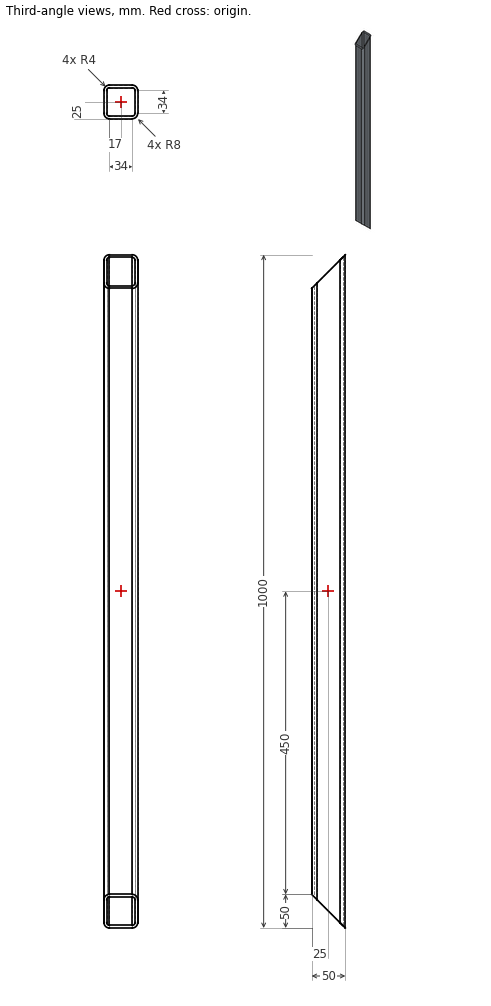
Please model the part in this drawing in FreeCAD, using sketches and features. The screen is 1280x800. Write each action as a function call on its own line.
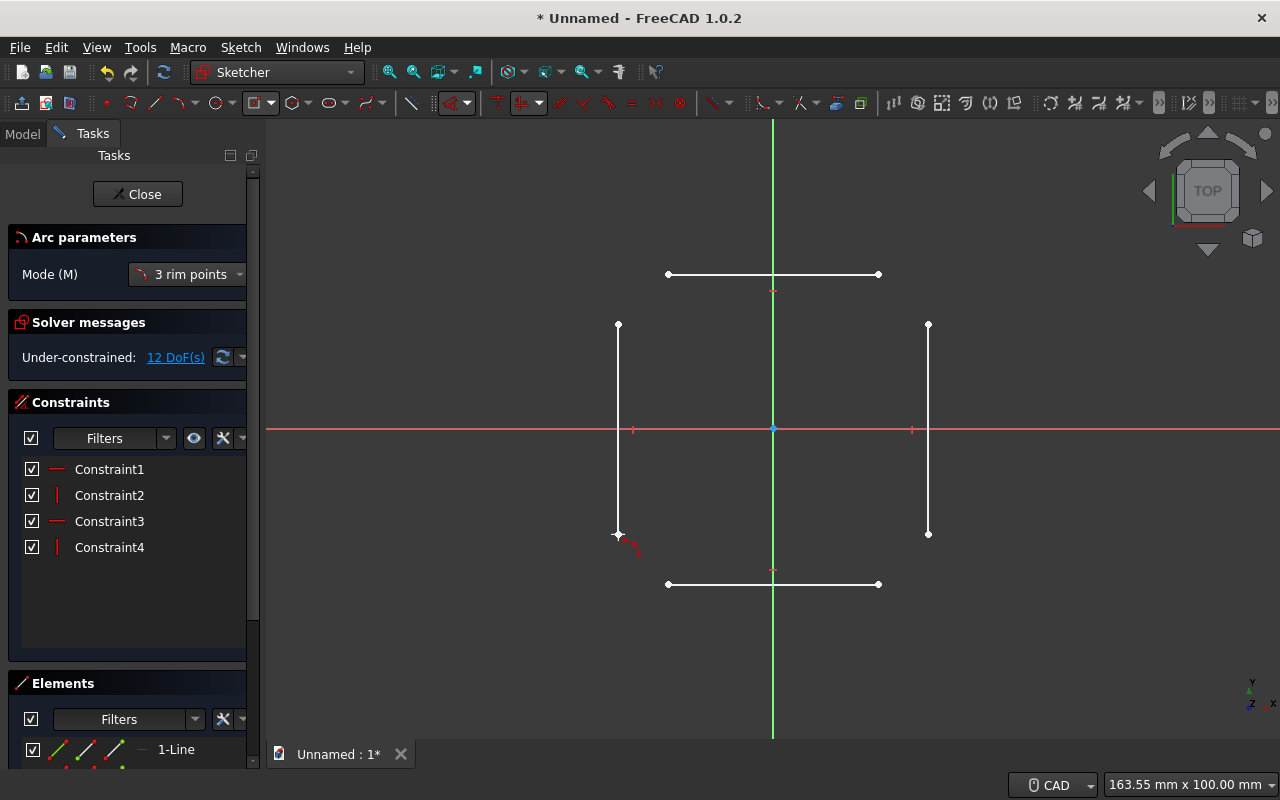
click(878, 585)
click(928, 535)
click(913, 569)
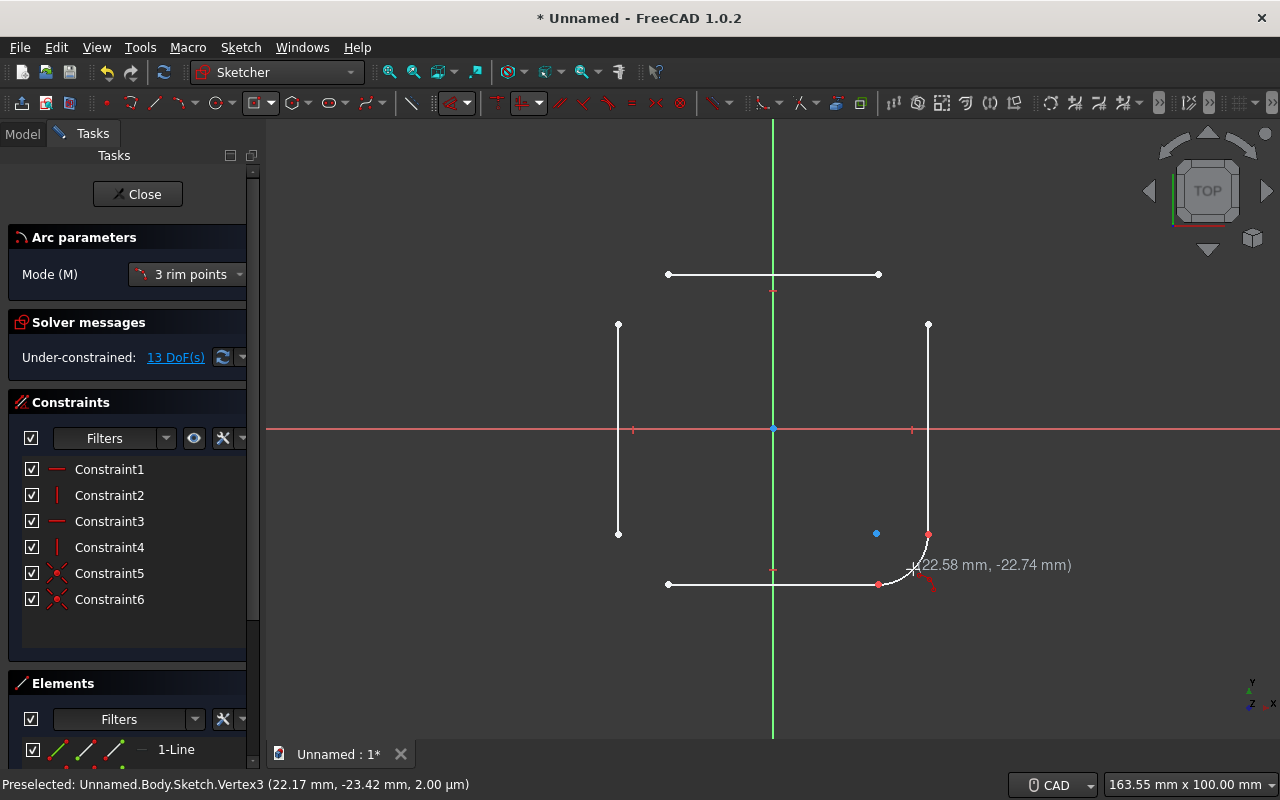
click(928, 325)
click(878, 275)
click(913, 289)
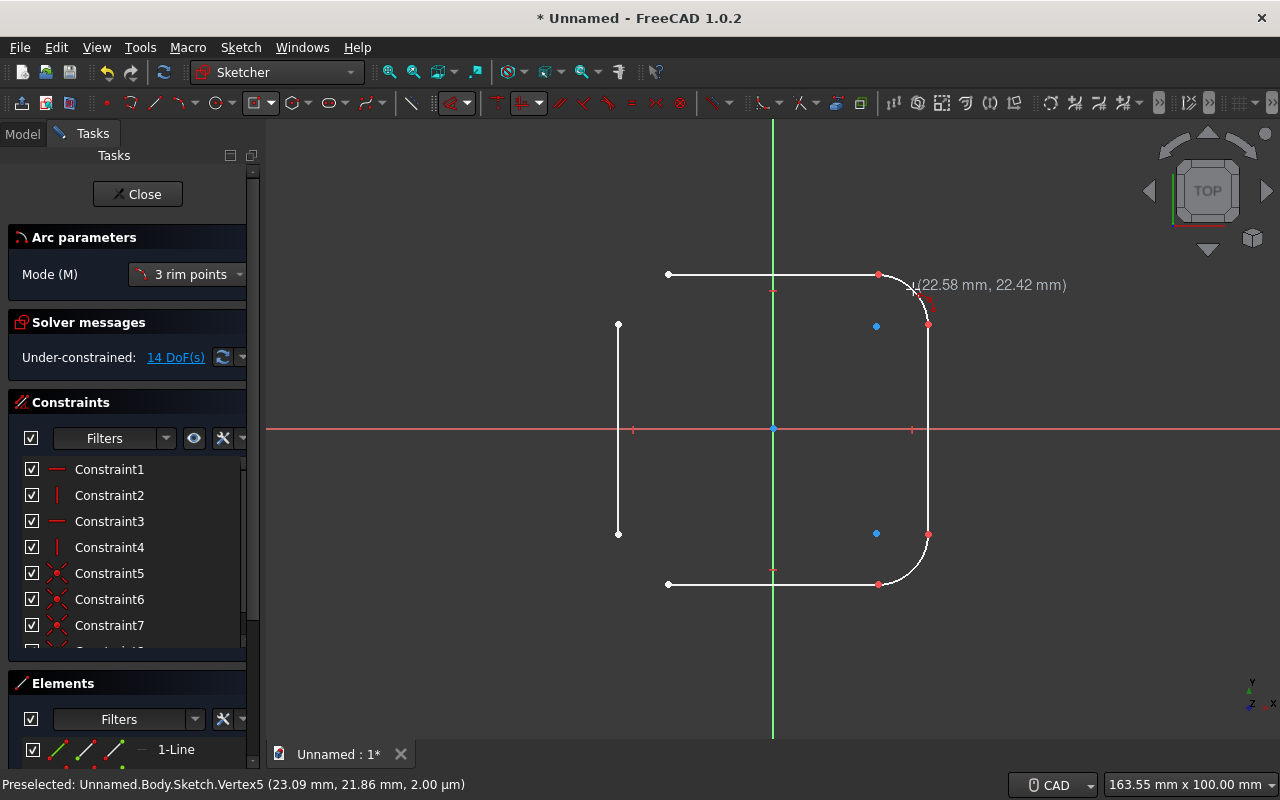
click(668, 275)
click(618, 325)
click(633, 289)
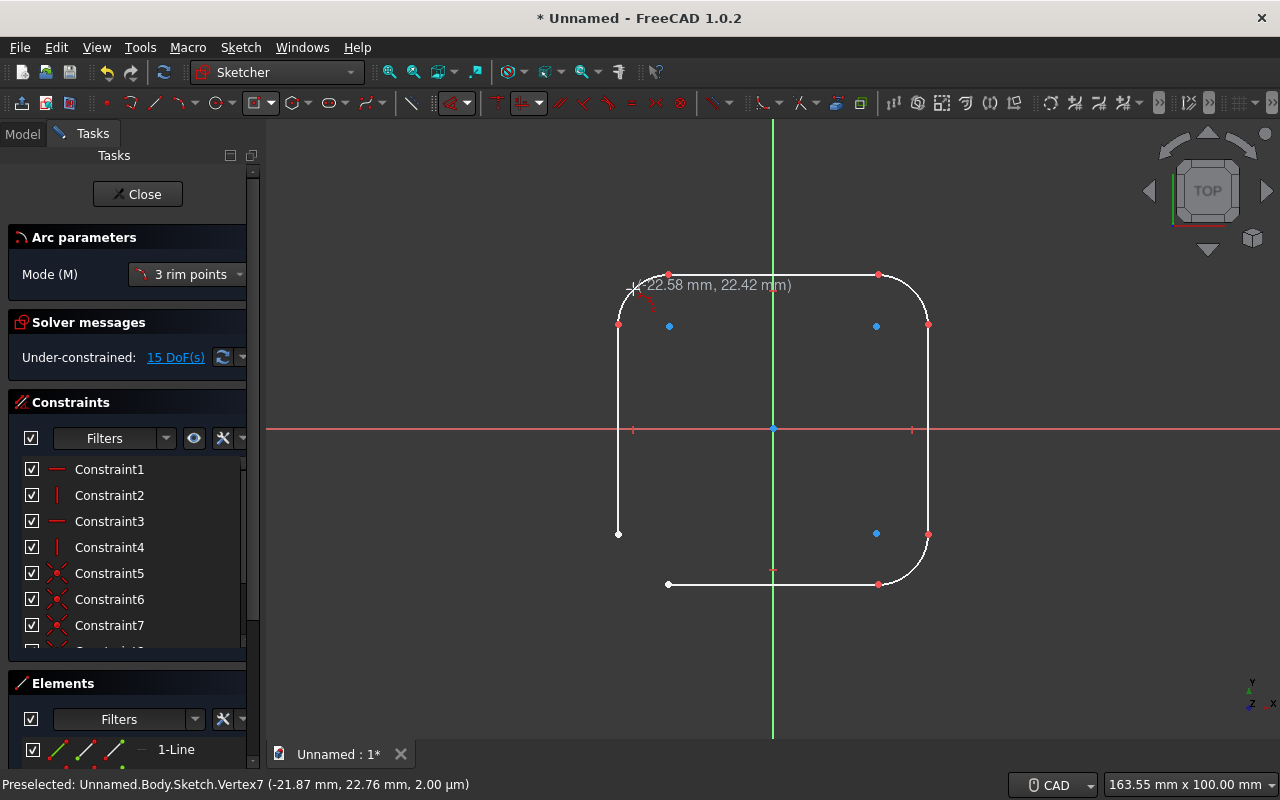
click(618, 535)
click(668, 585)
click(633, 569)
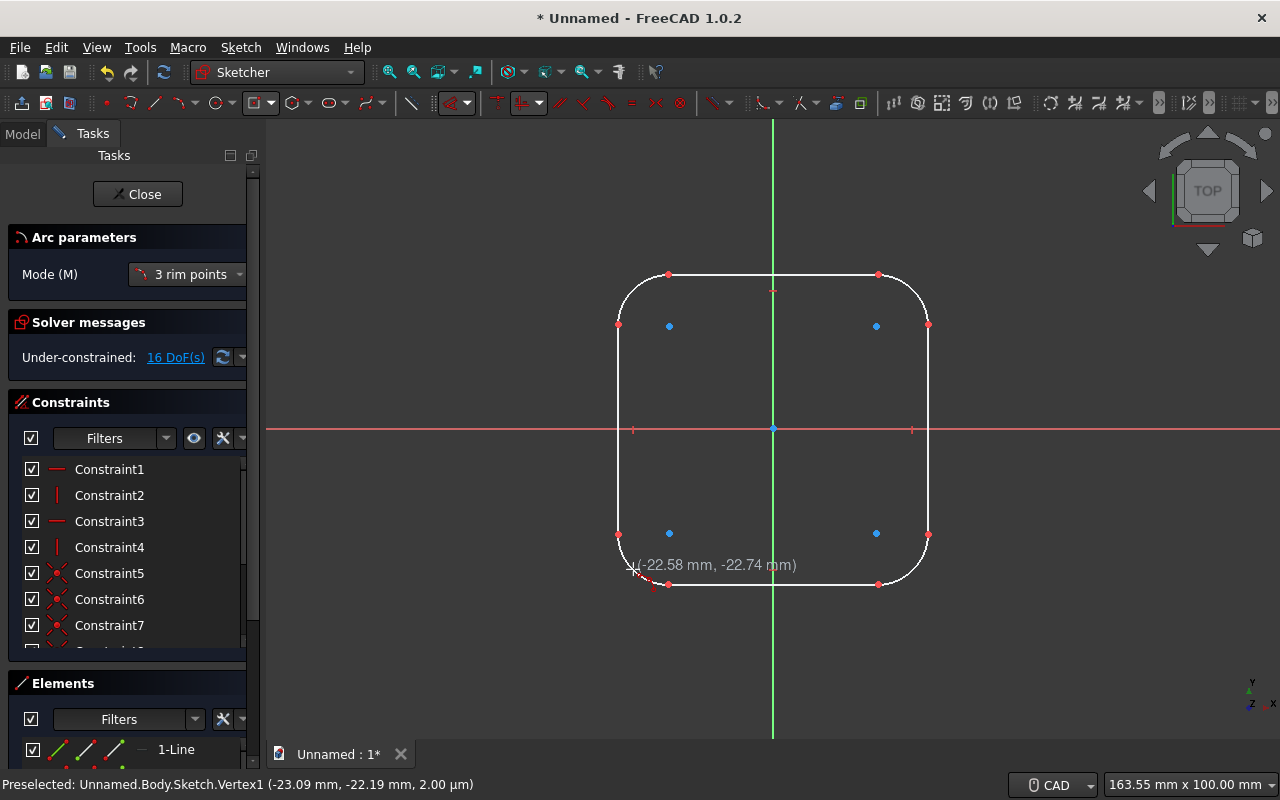
key(g)
key(l)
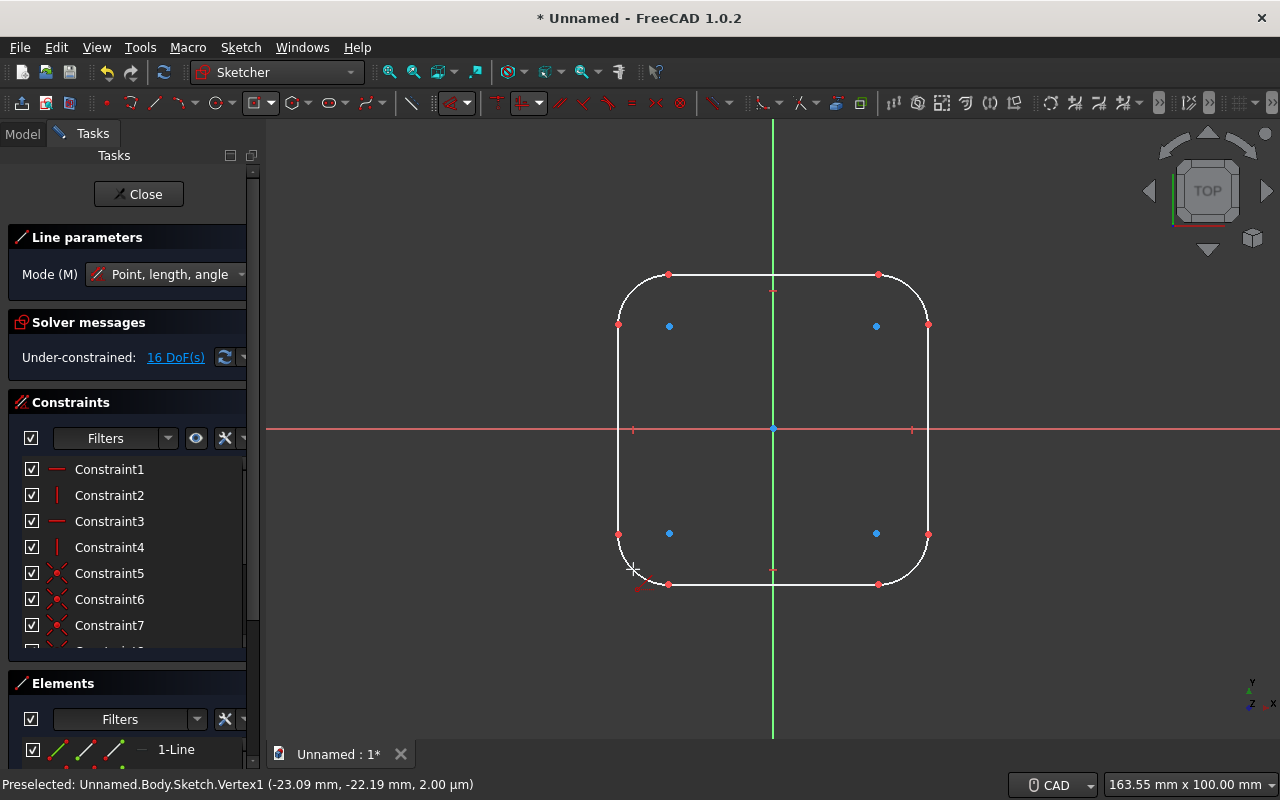
click(668, 299)
click(878, 299)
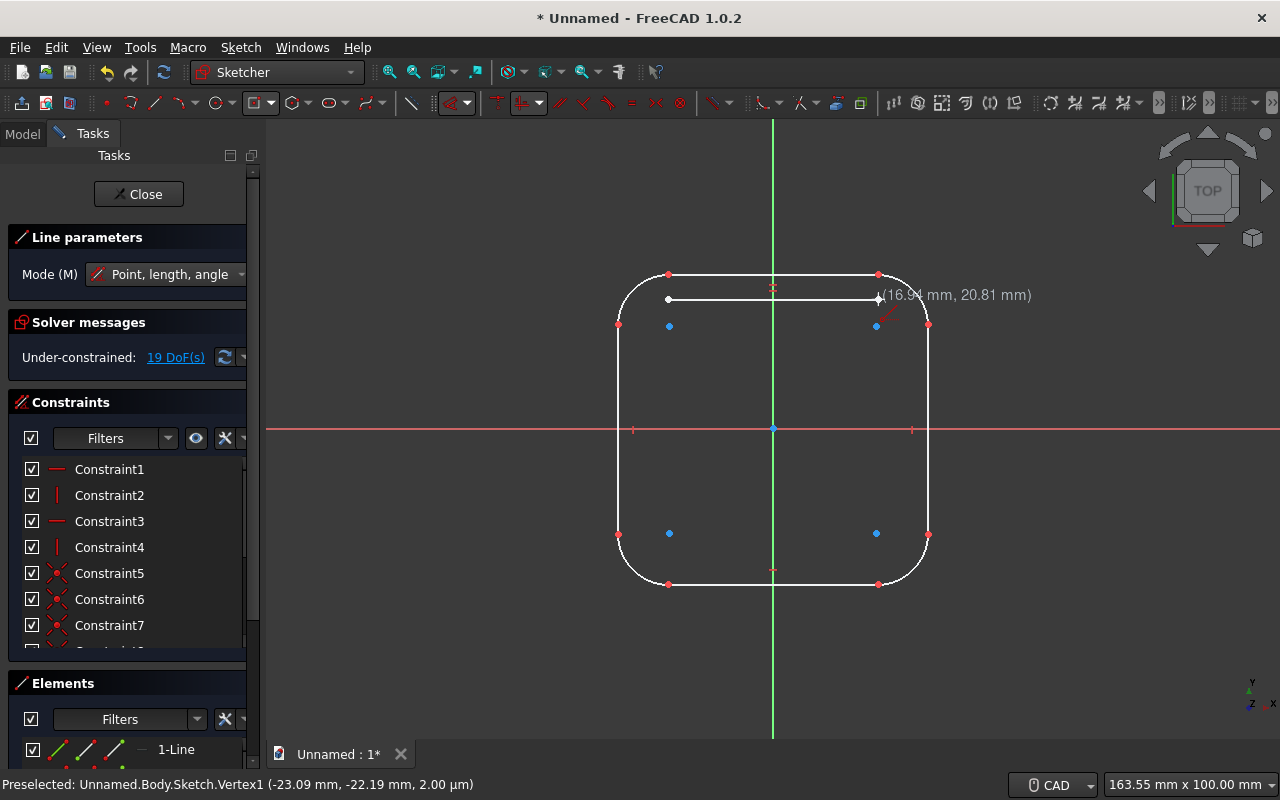
click(903, 324)
click(903, 534)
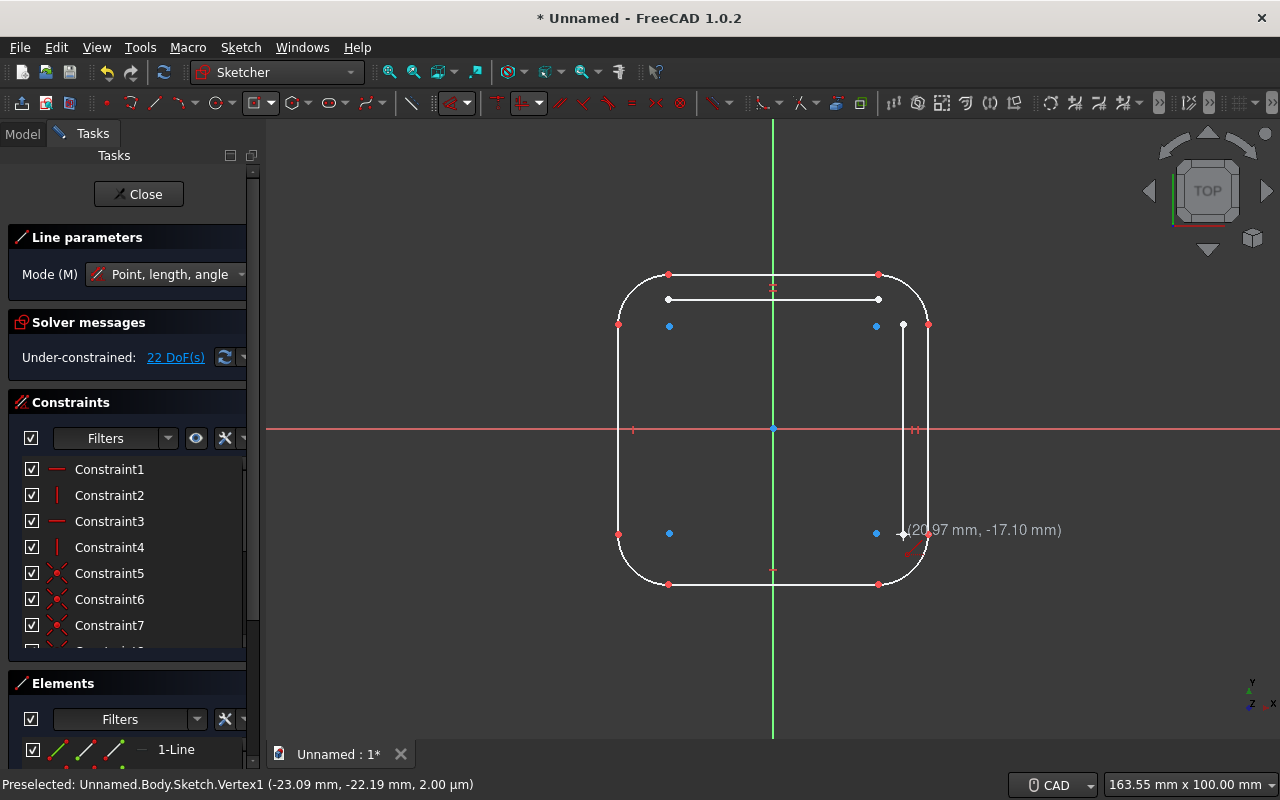
click(878, 559)
click(668, 559)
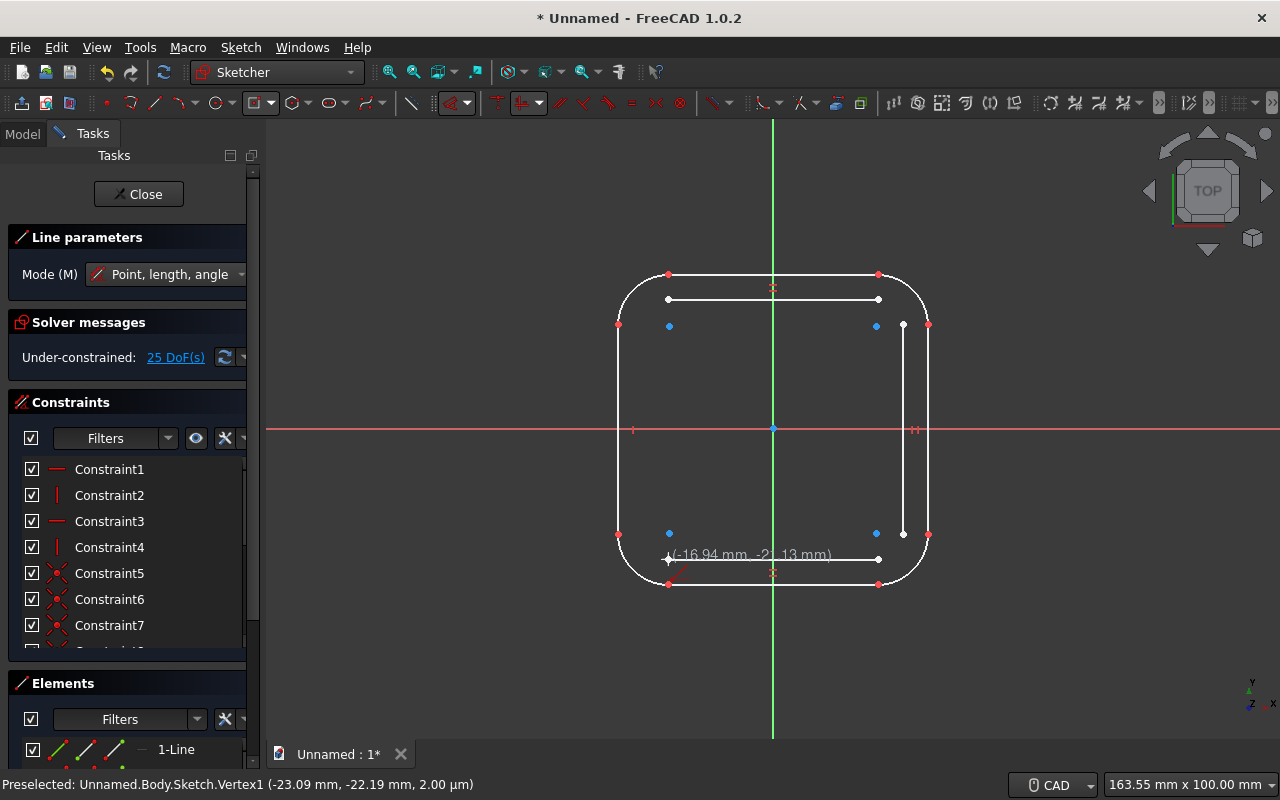
click(643, 534)
click(643, 324)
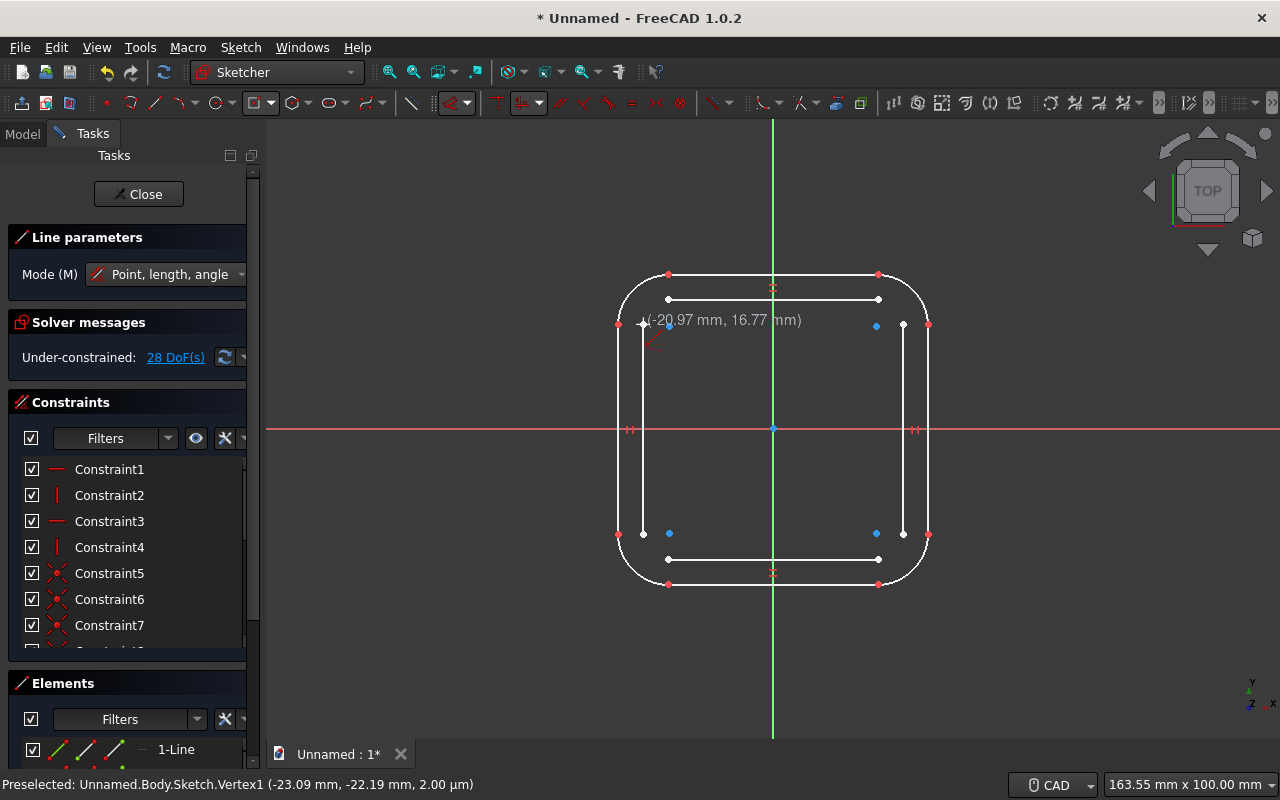
key(g)
key(3)
key(a)